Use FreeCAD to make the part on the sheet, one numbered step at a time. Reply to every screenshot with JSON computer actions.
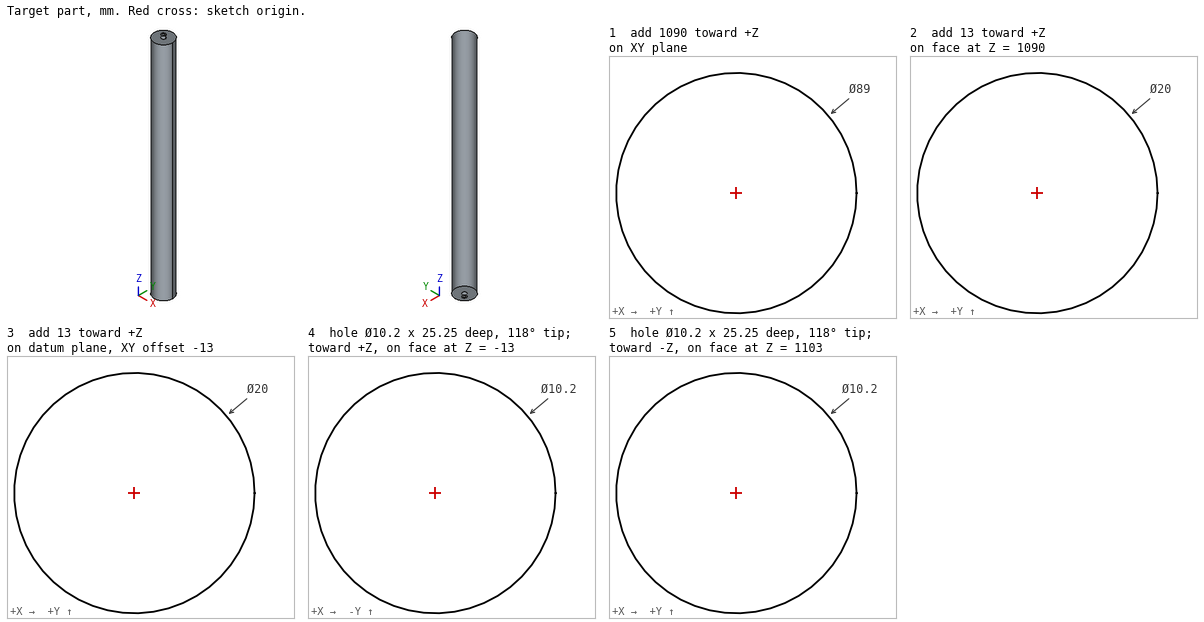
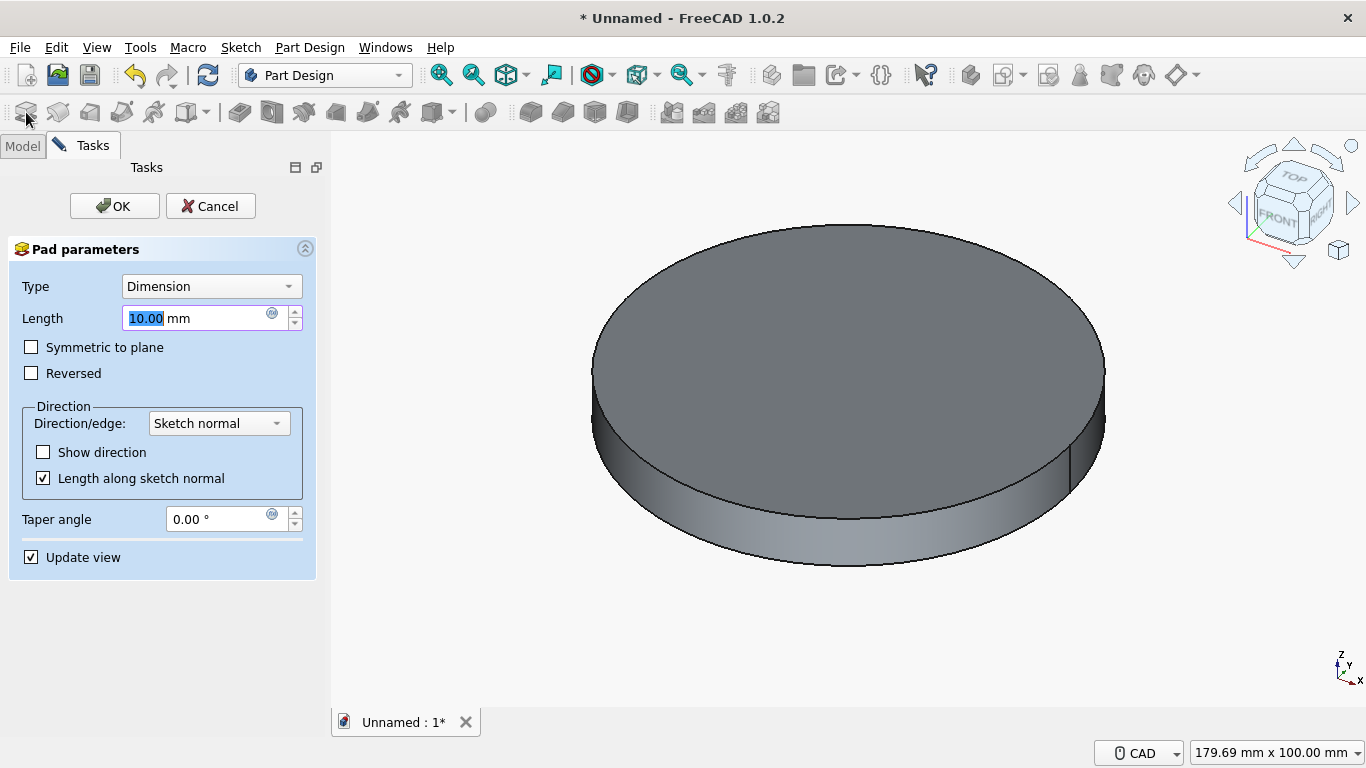
{"action": "type", "text": "1090"}
{"action": "key", "text": "Tab"}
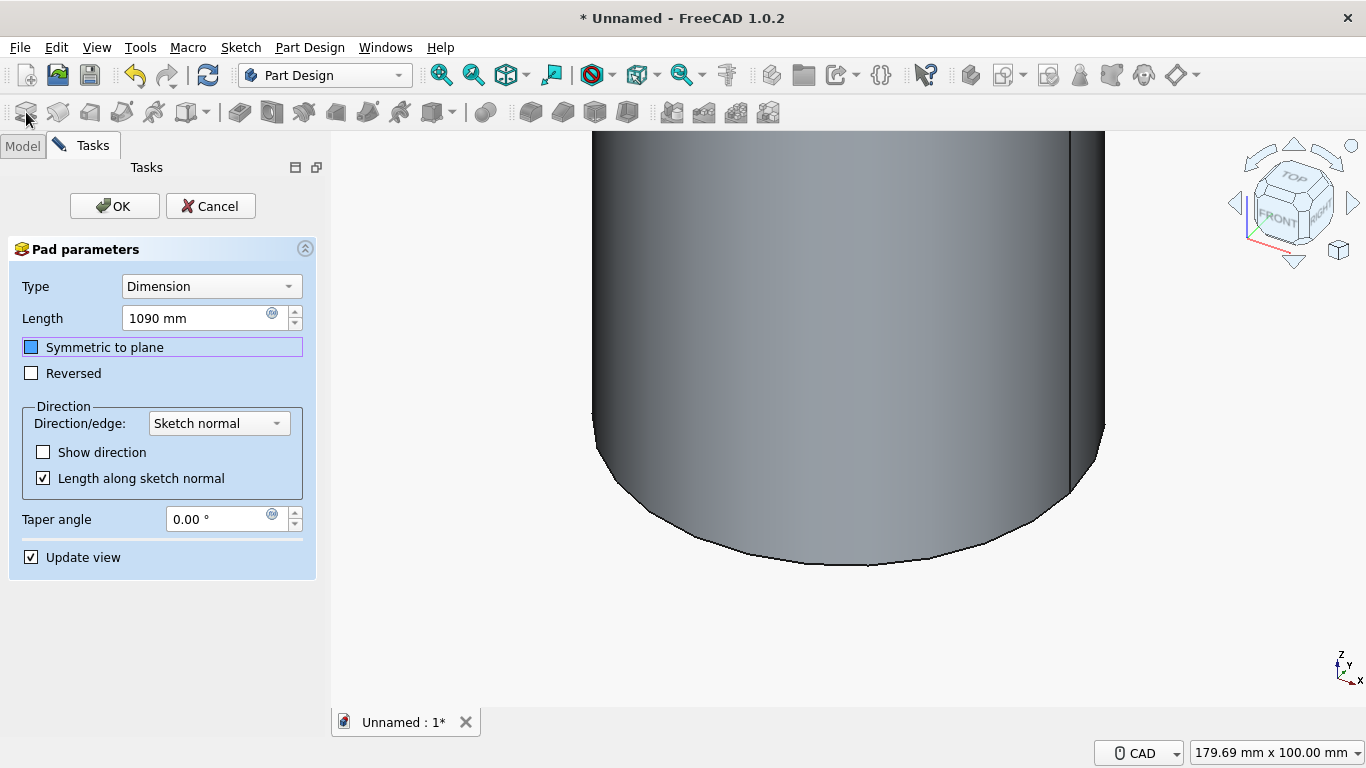
{"action": "left_click", "coordinate": [115, 206]}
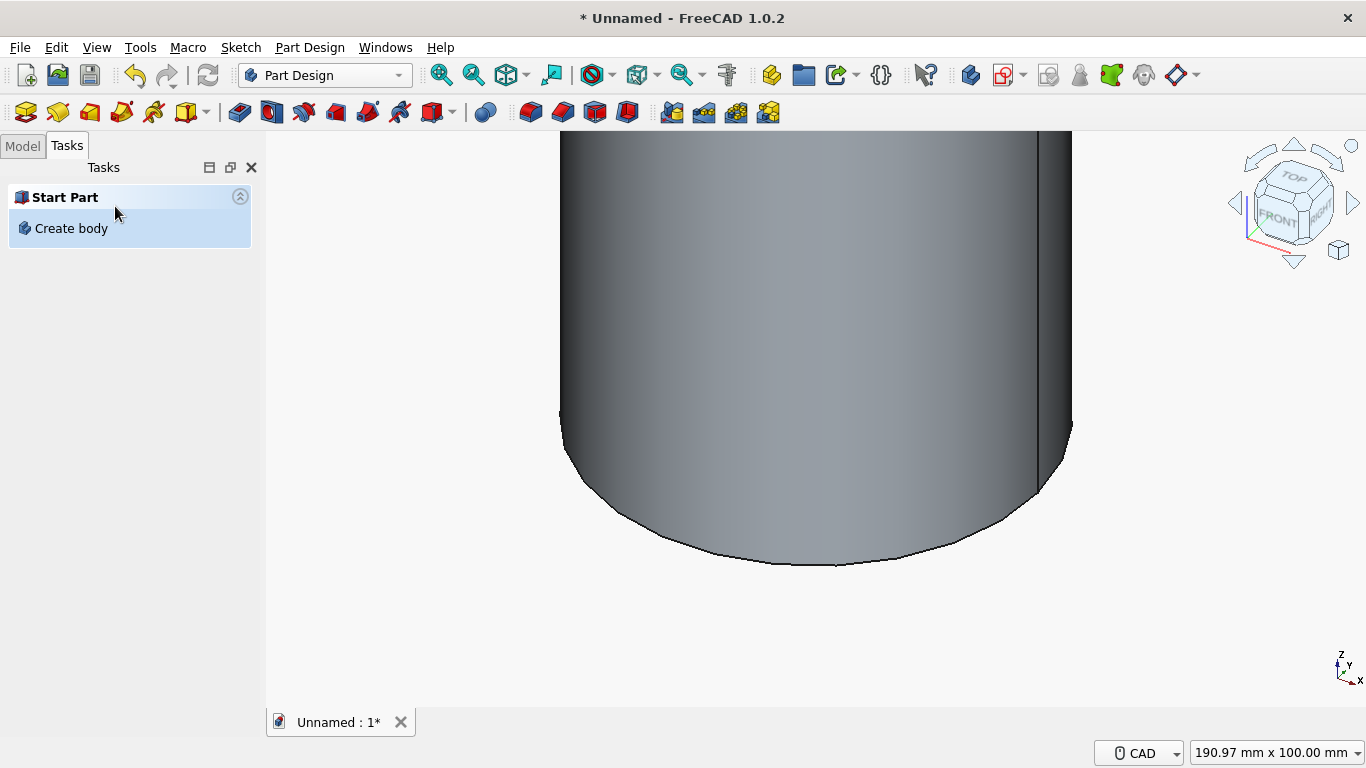
{"action": "key", "text": "v f"}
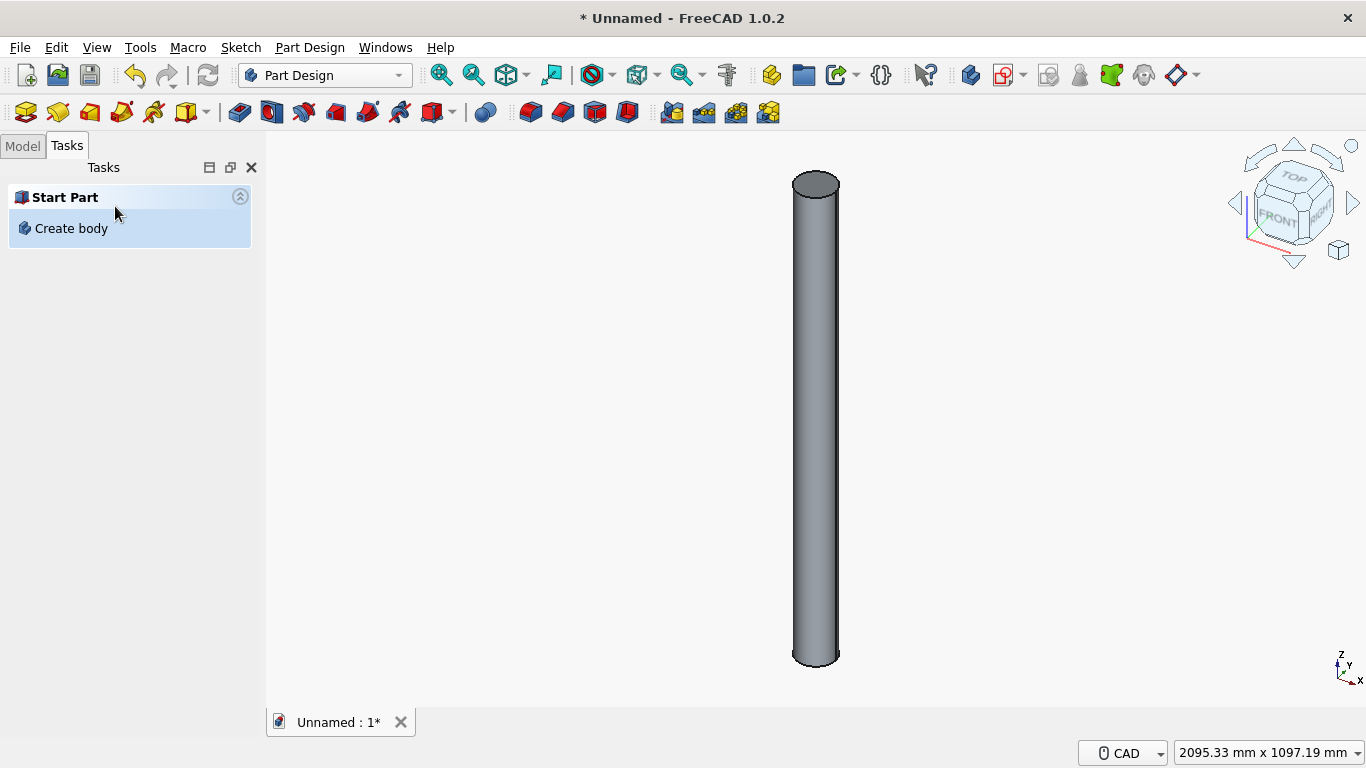
{"action": "left_click", "coordinate": [816, 184]}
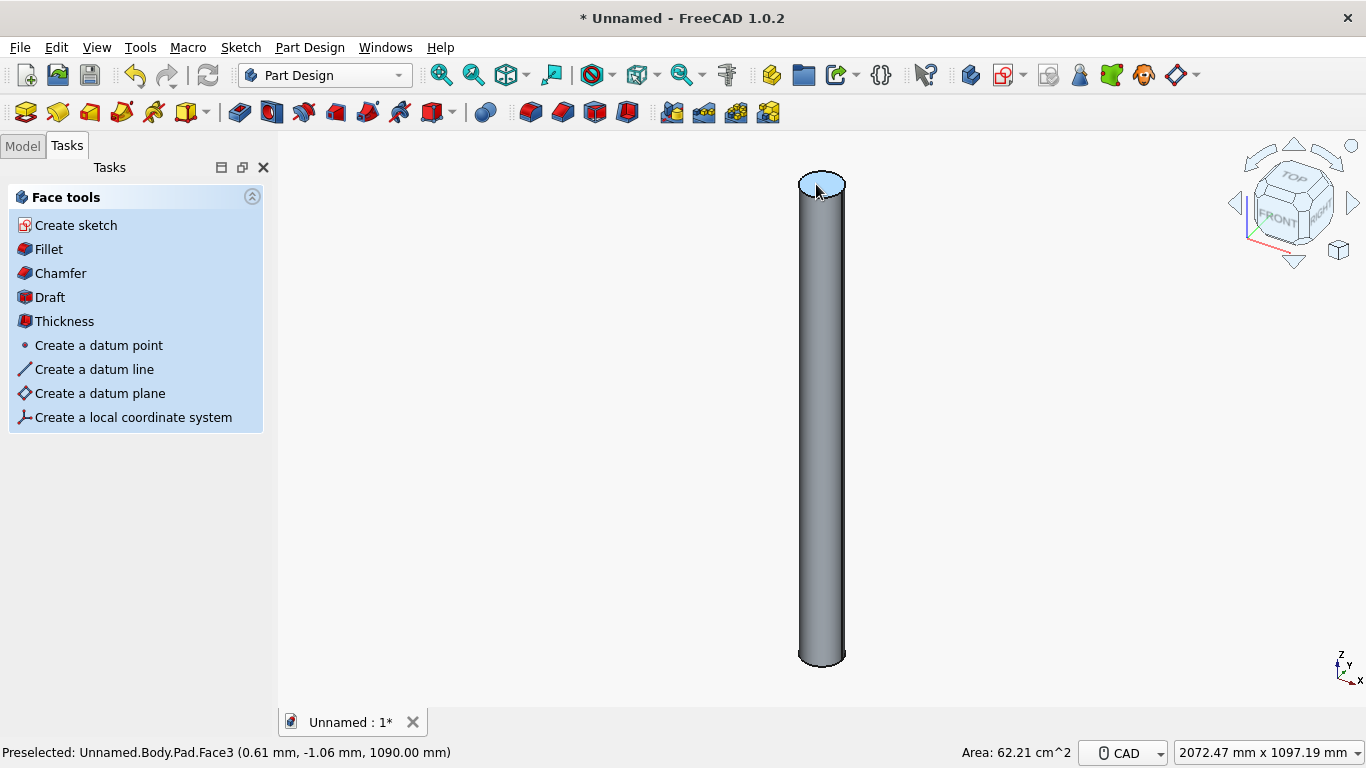
{"action": "left_click", "coordinate": [1004, 76]}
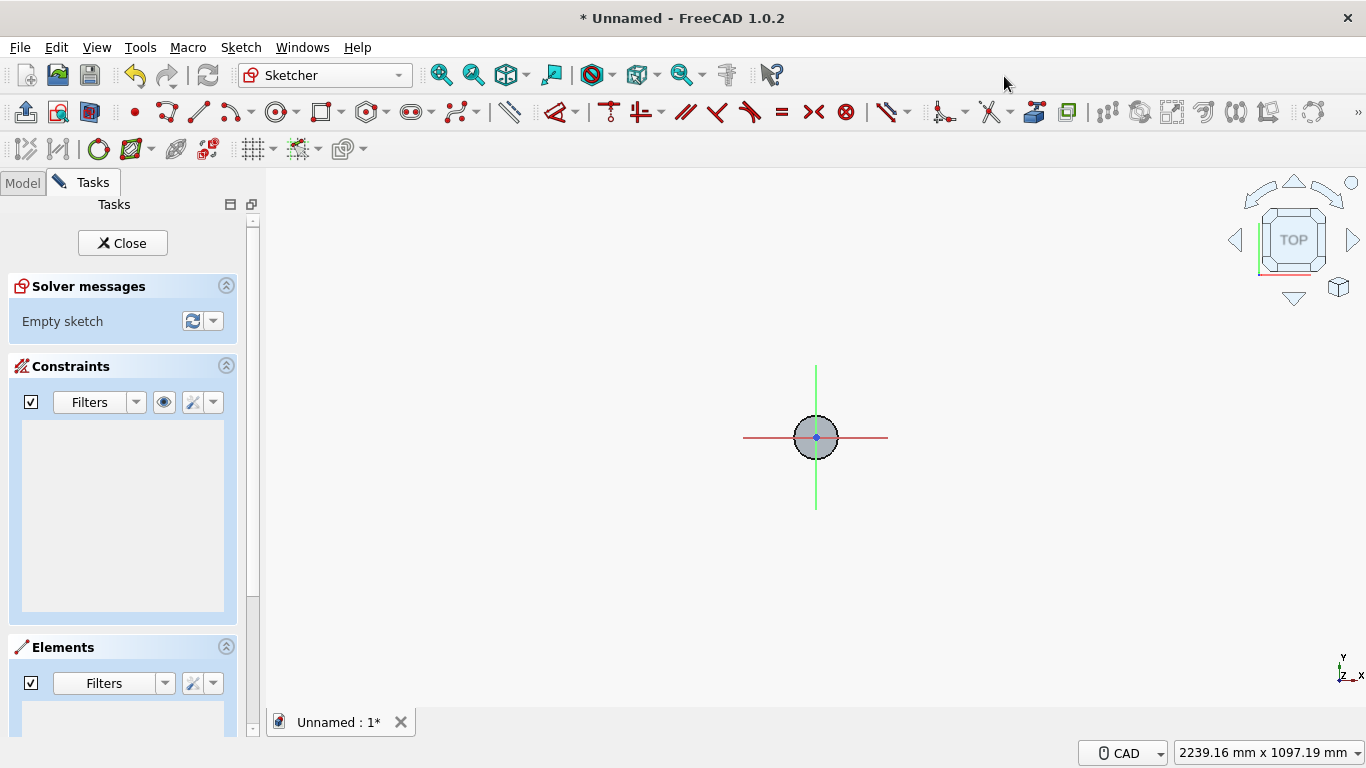
{"action": "scroll", "coordinate": [820, 438], "scroll_direction": "up", "scroll_amount": 15}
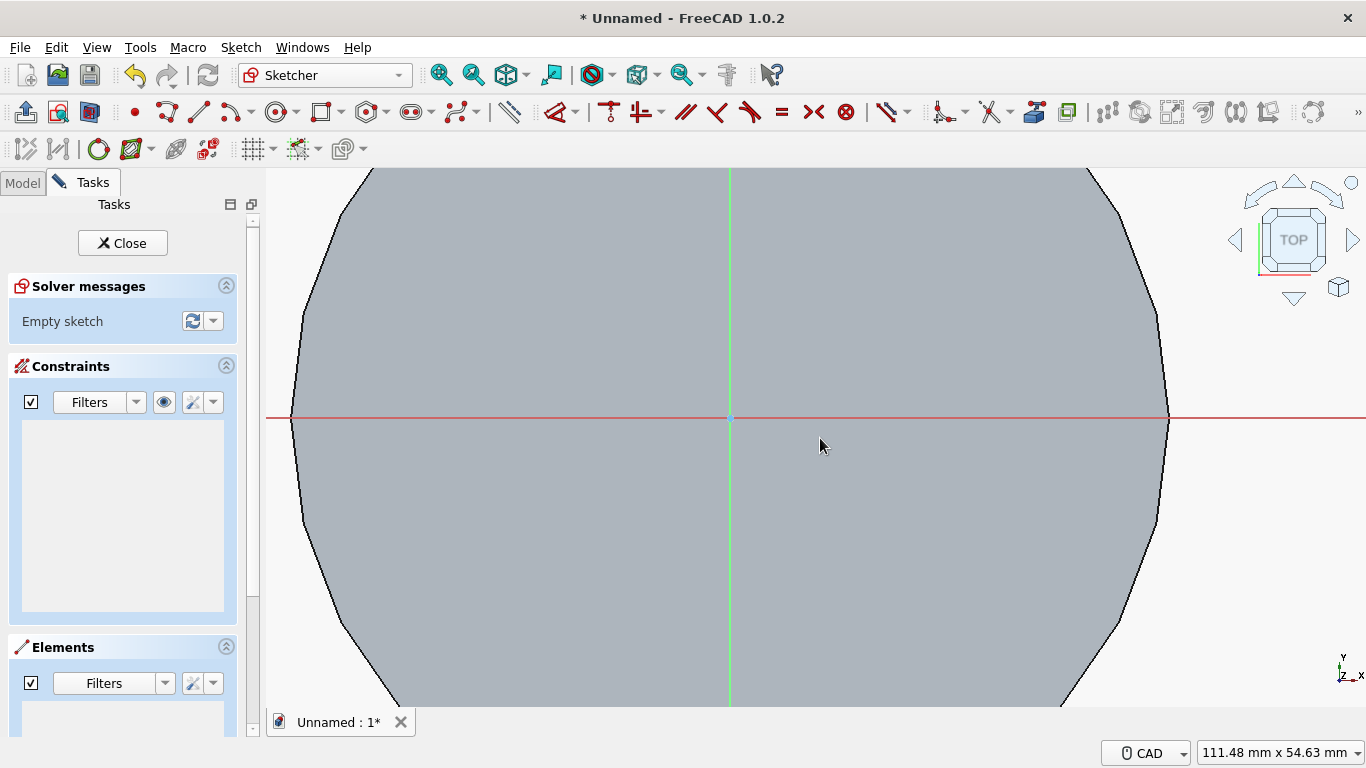
{"action": "scroll", "coordinate": [709, 395], "scroll_direction": "up", "scroll_amount": 3}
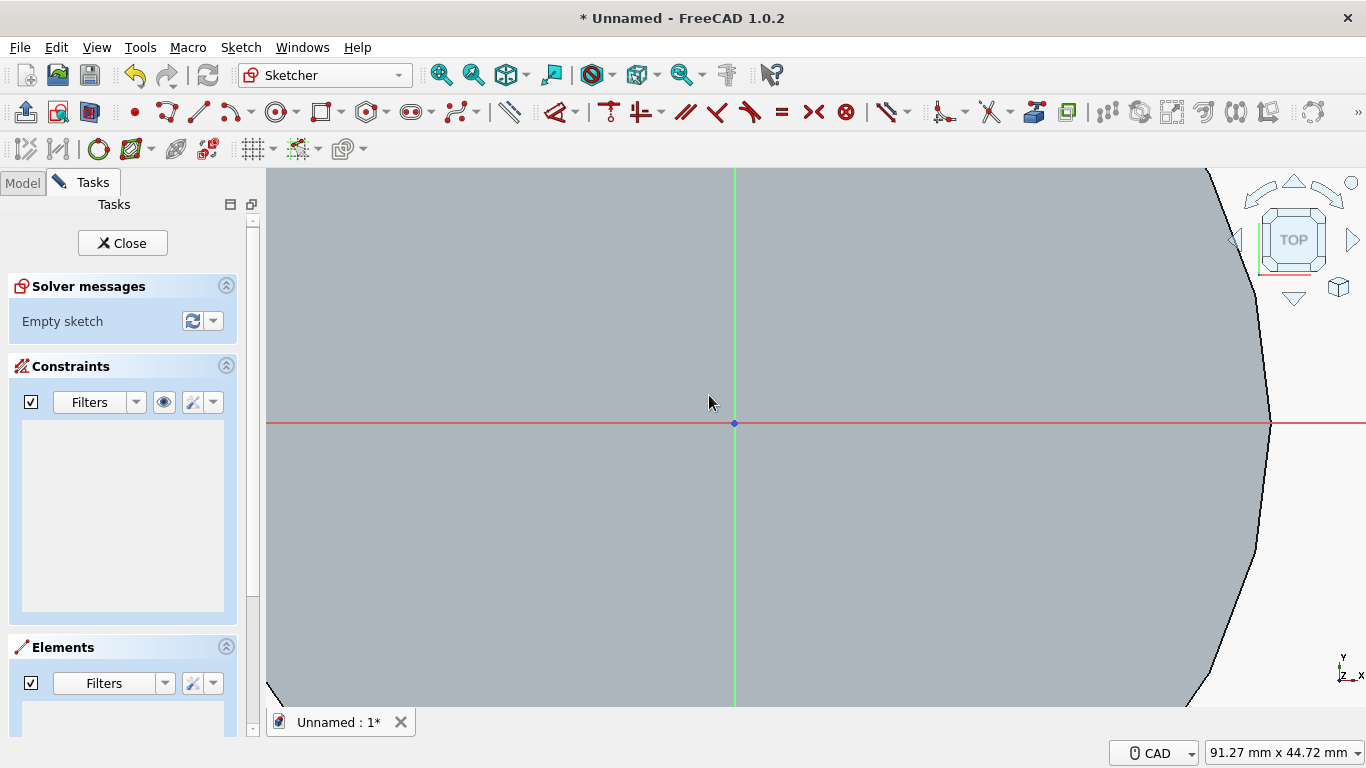
{"action": "left_click", "coordinate": [276, 112]}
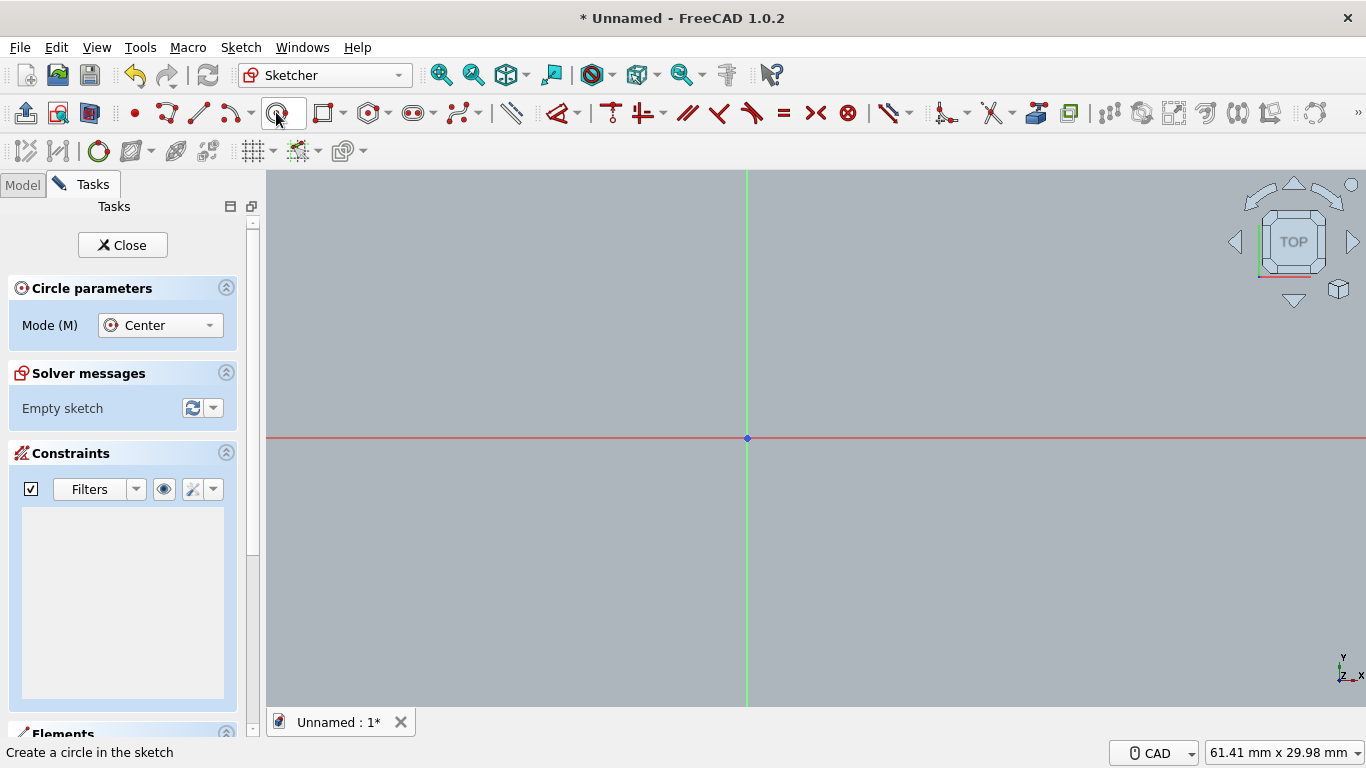
{"action": "left_click", "coordinate": [747, 438]}
{"action": "mouse_move", "coordinate": [874, 312]}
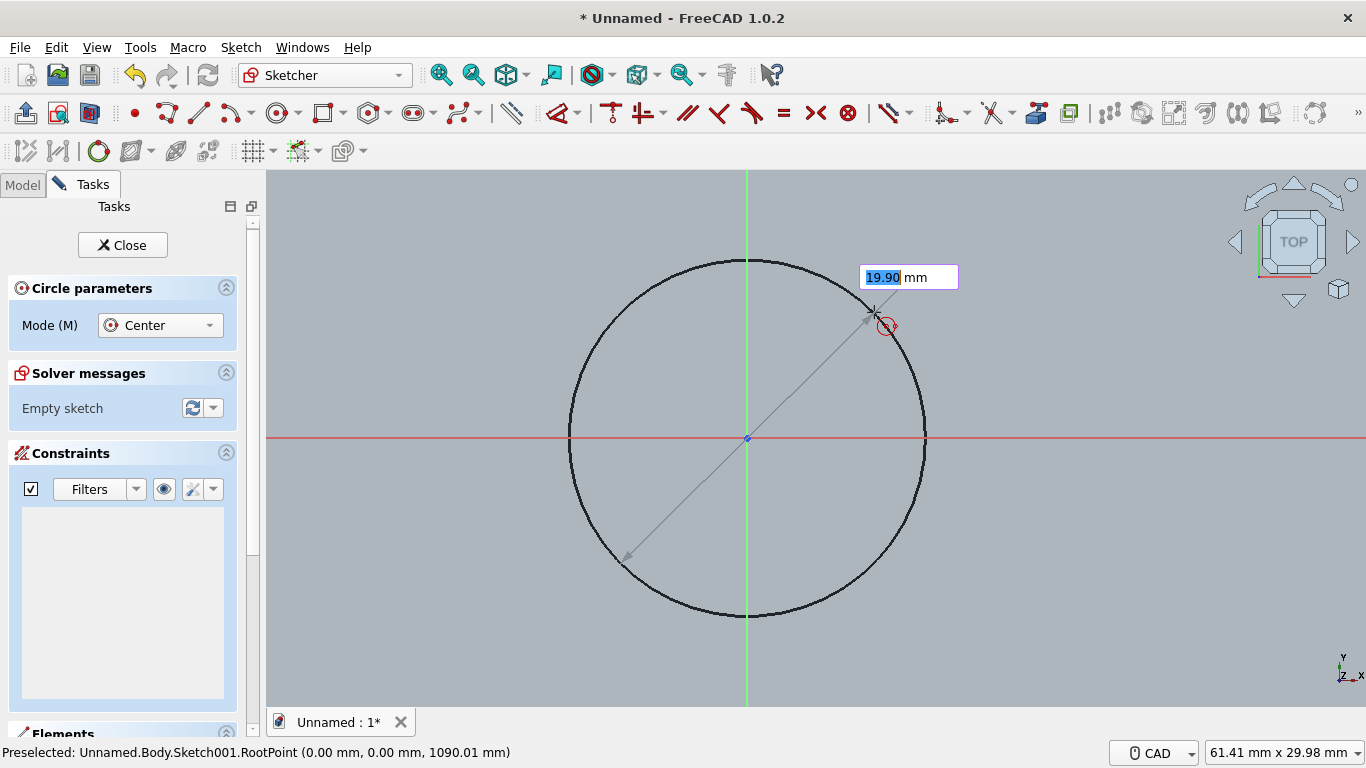
{"action": "type", "text": "20"}
{"action": "key", "text": "Return"}
{"action": "key", "text": "Escape"}